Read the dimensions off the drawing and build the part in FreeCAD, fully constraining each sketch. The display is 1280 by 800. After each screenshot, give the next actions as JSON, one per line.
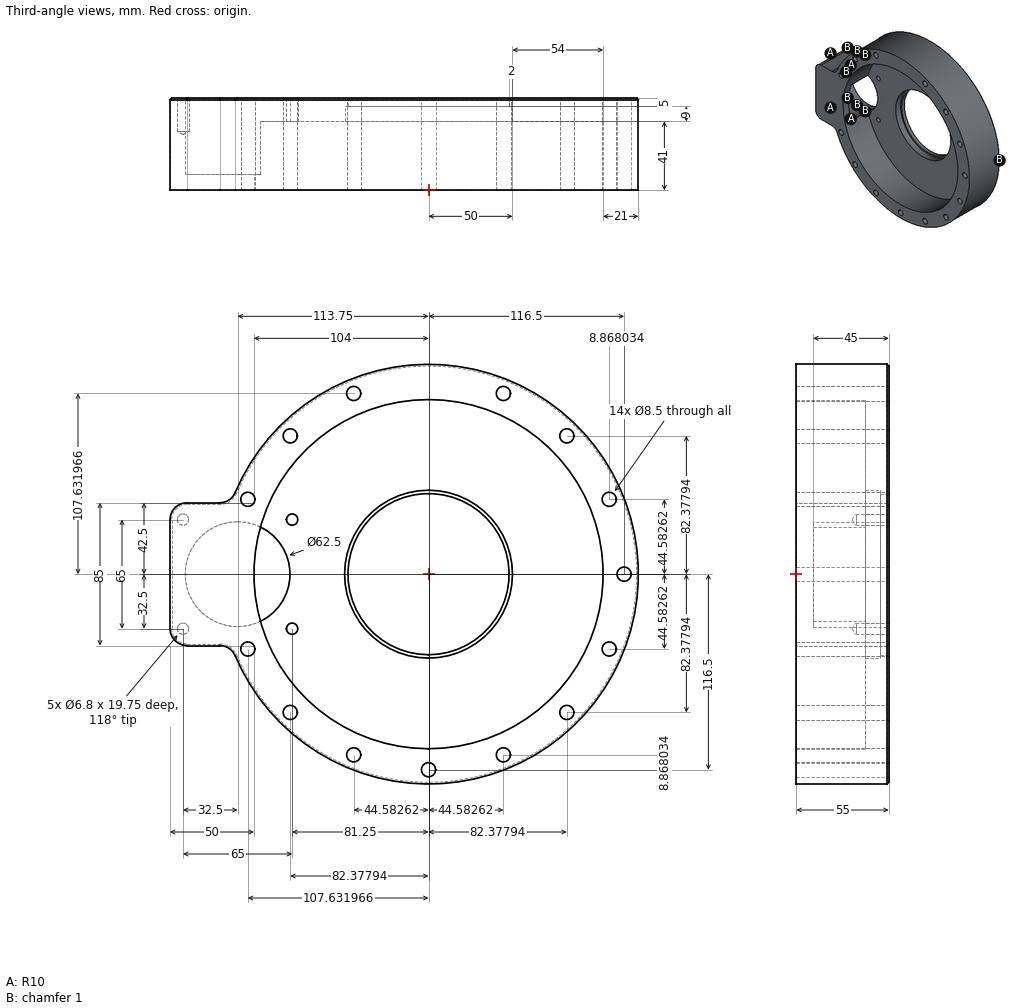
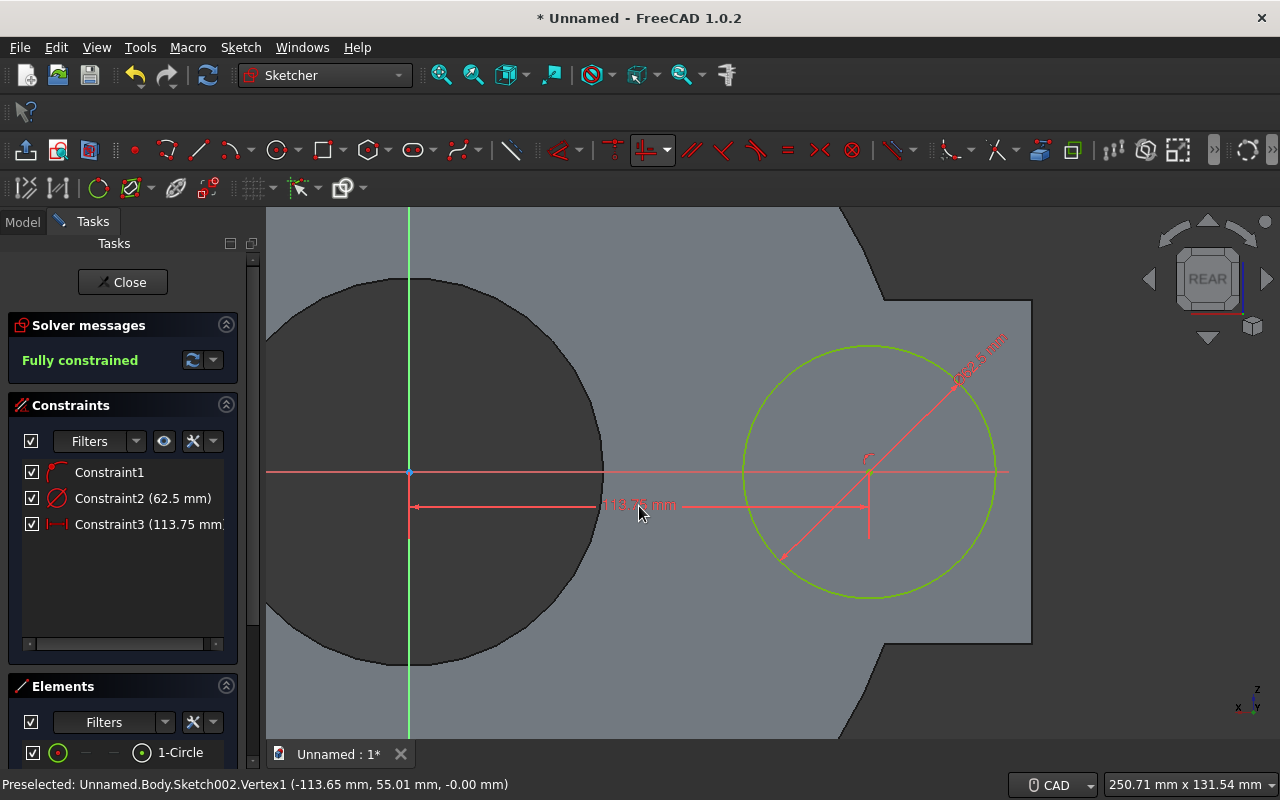
{"action": "left_click", "coordinate": [123, 282]}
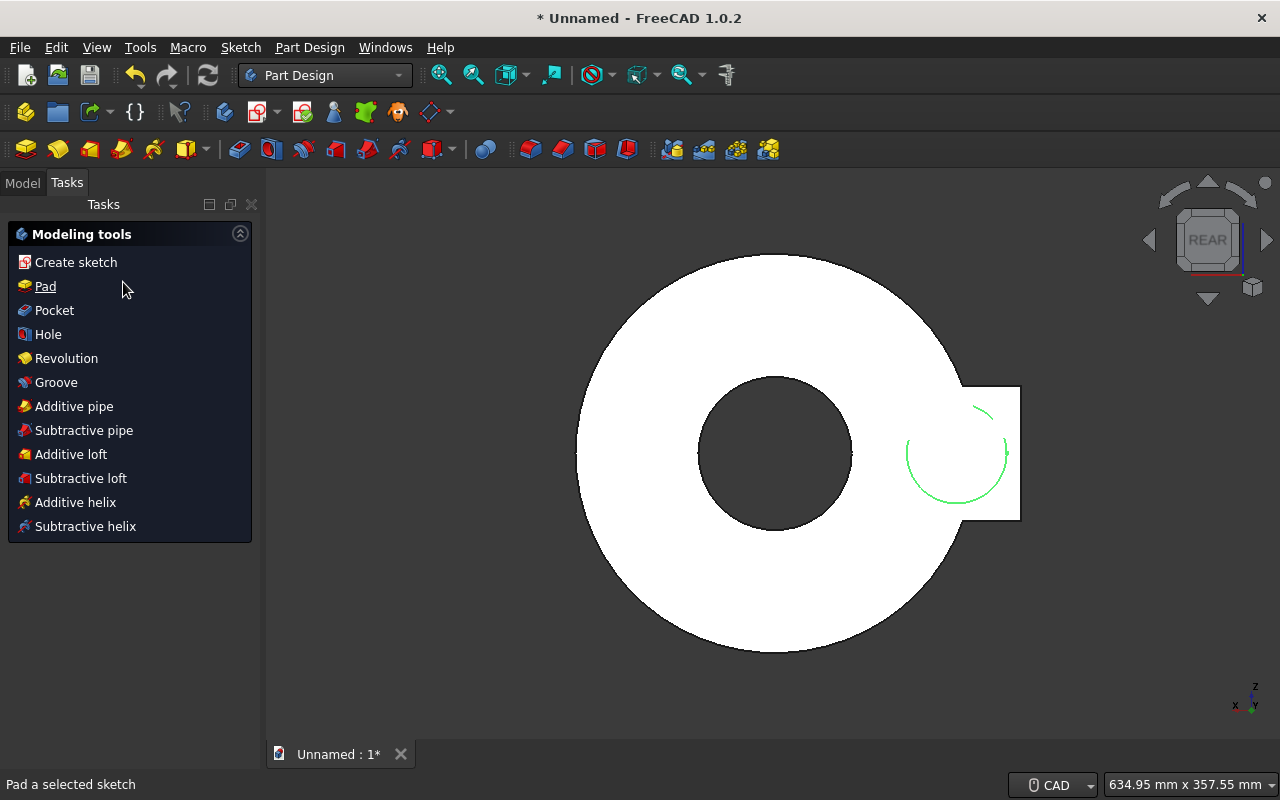
{"action": "left_click", "coordinate": [240, 150]}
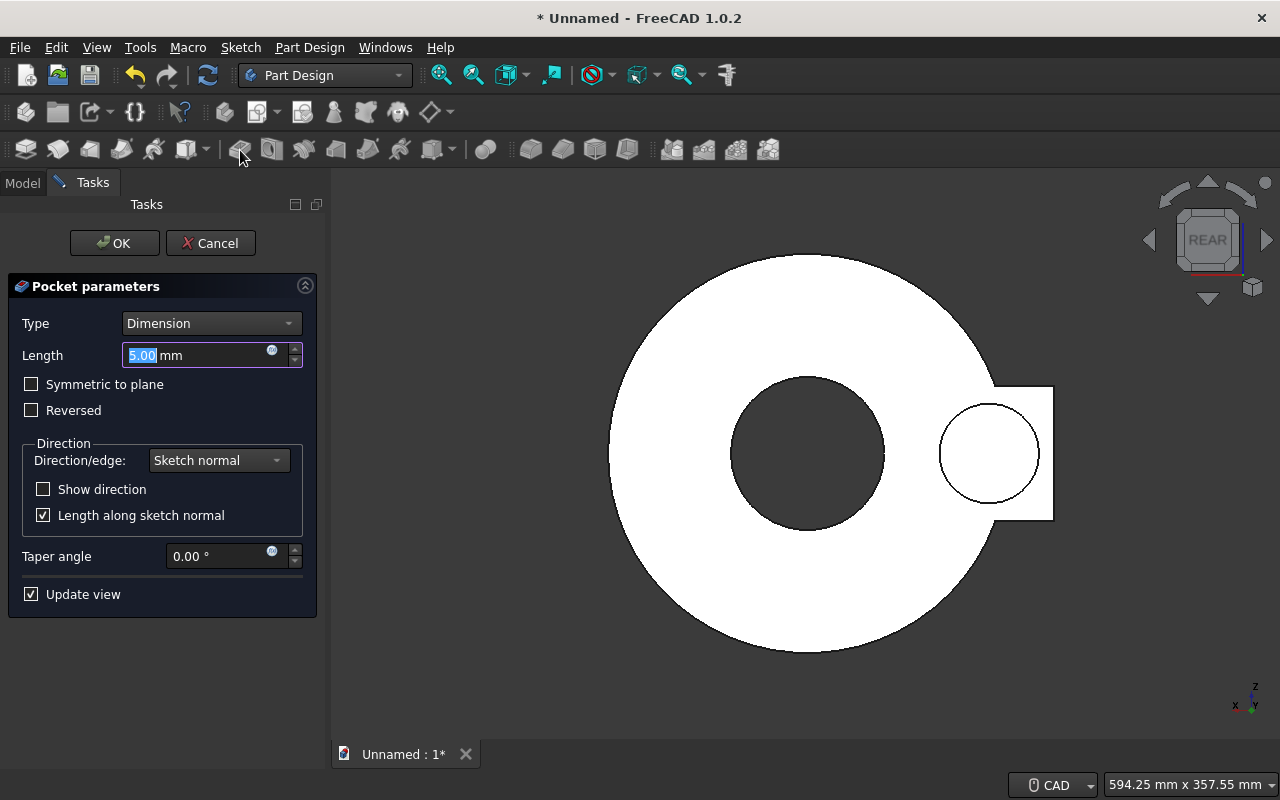
{"action": "type", "text": "45"}
{"action": "key", "text": "Tab"}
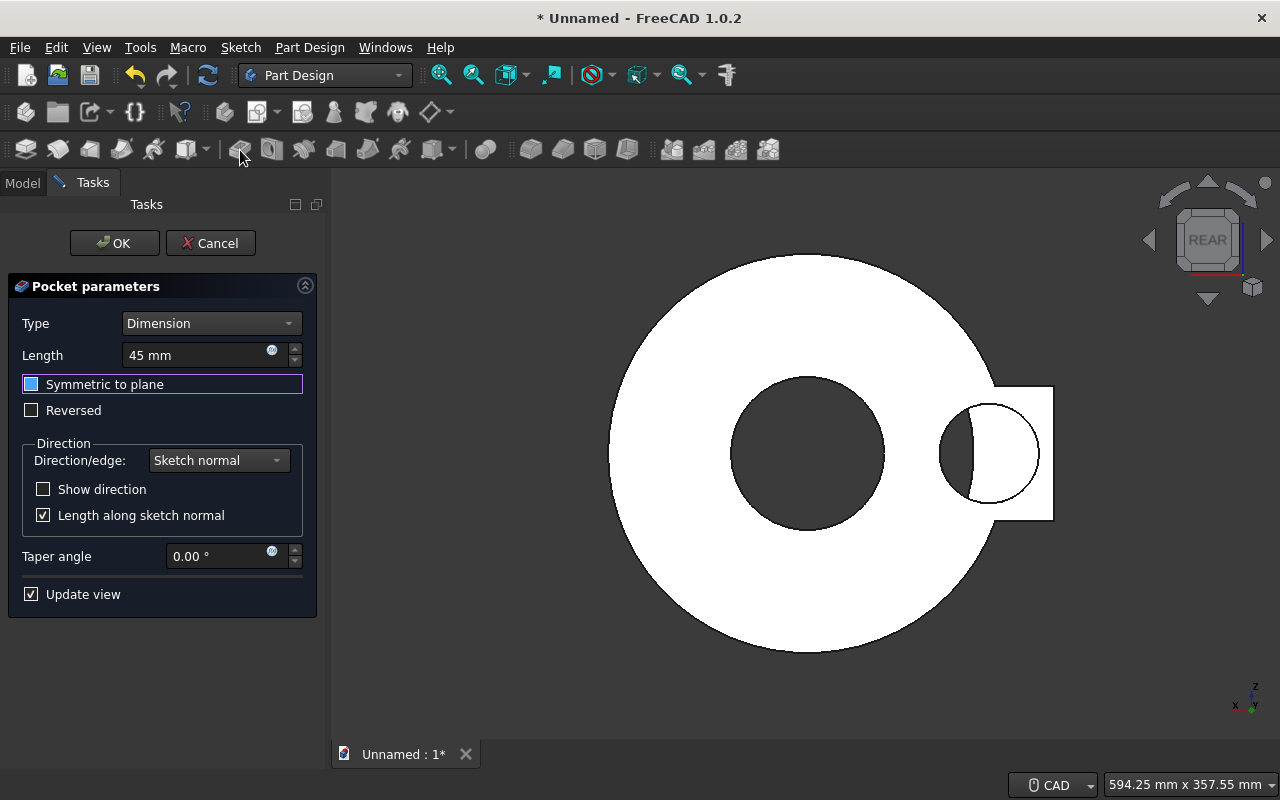
{"action": "left_click", "coordinate": [115, 243]}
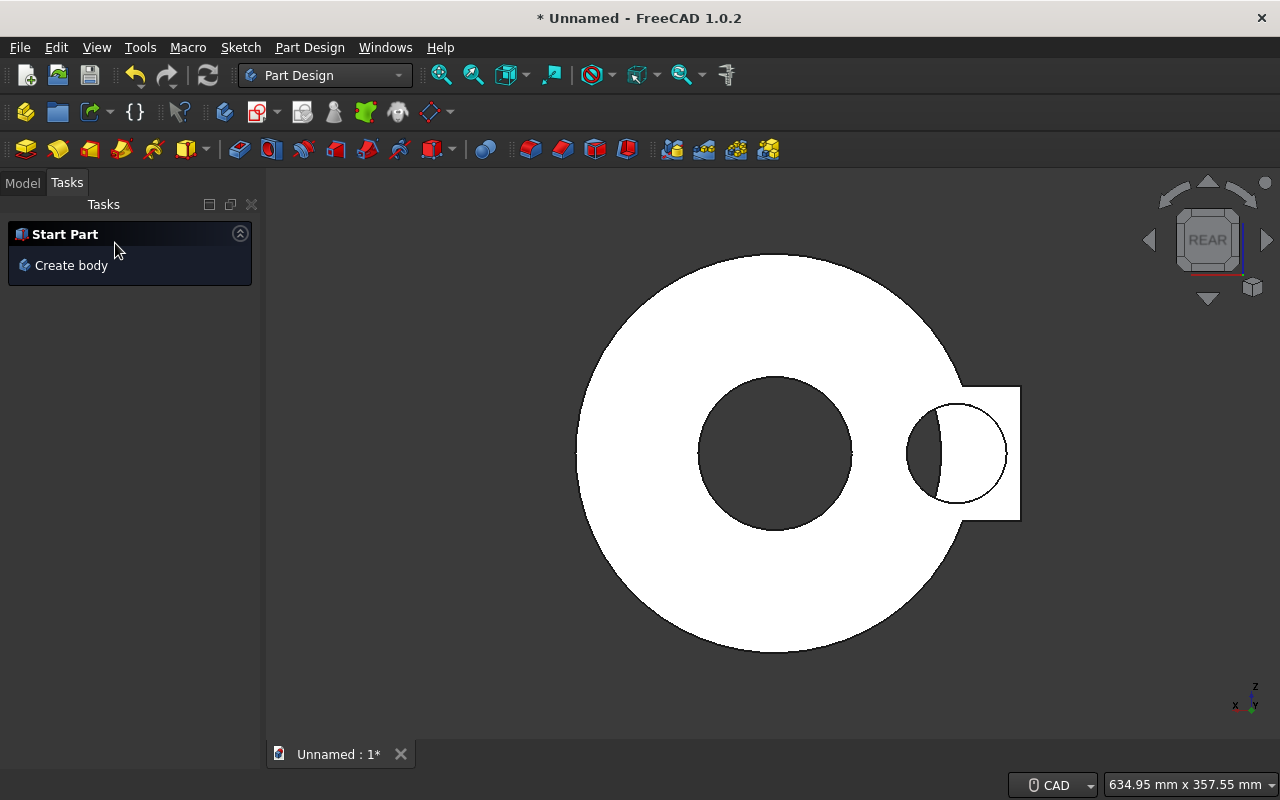
{"action": "left_click", "coordinate": [862, 338]}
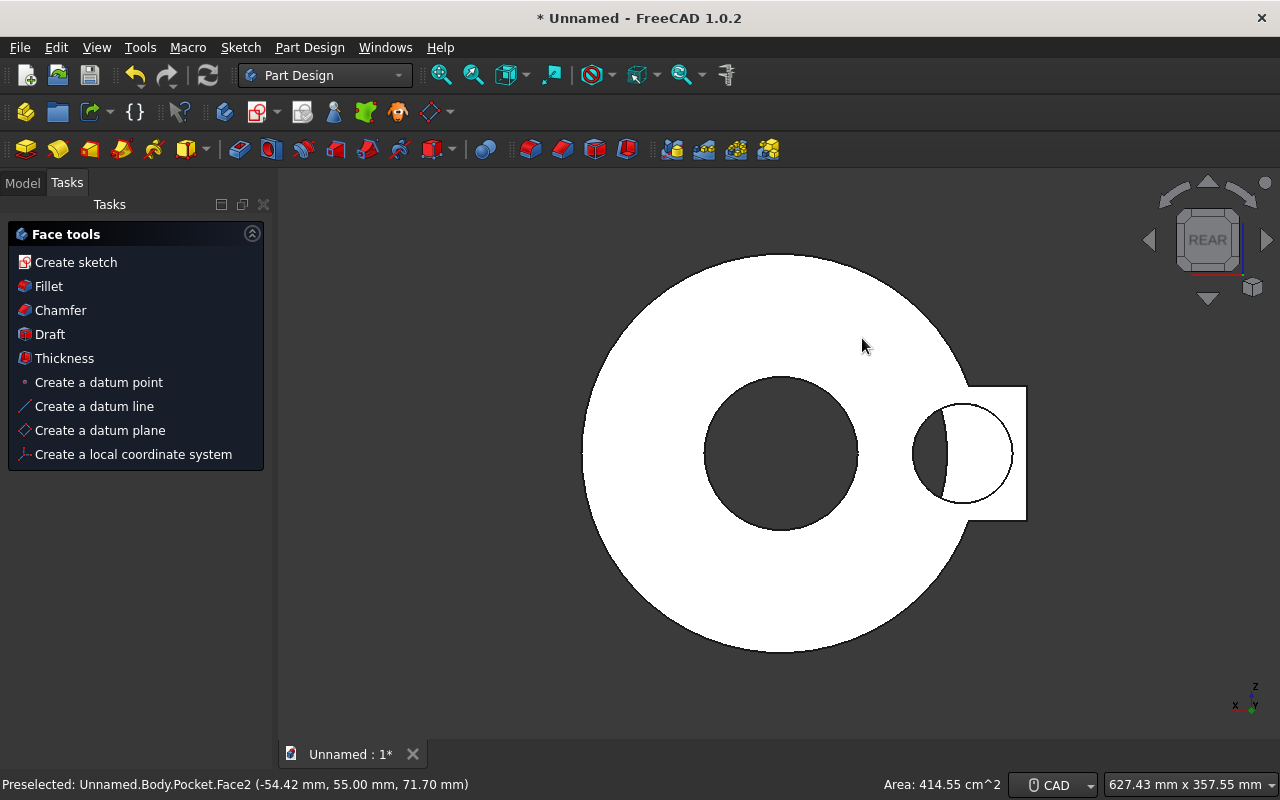
{"action": "left_click", "coordinate": [258, 112]}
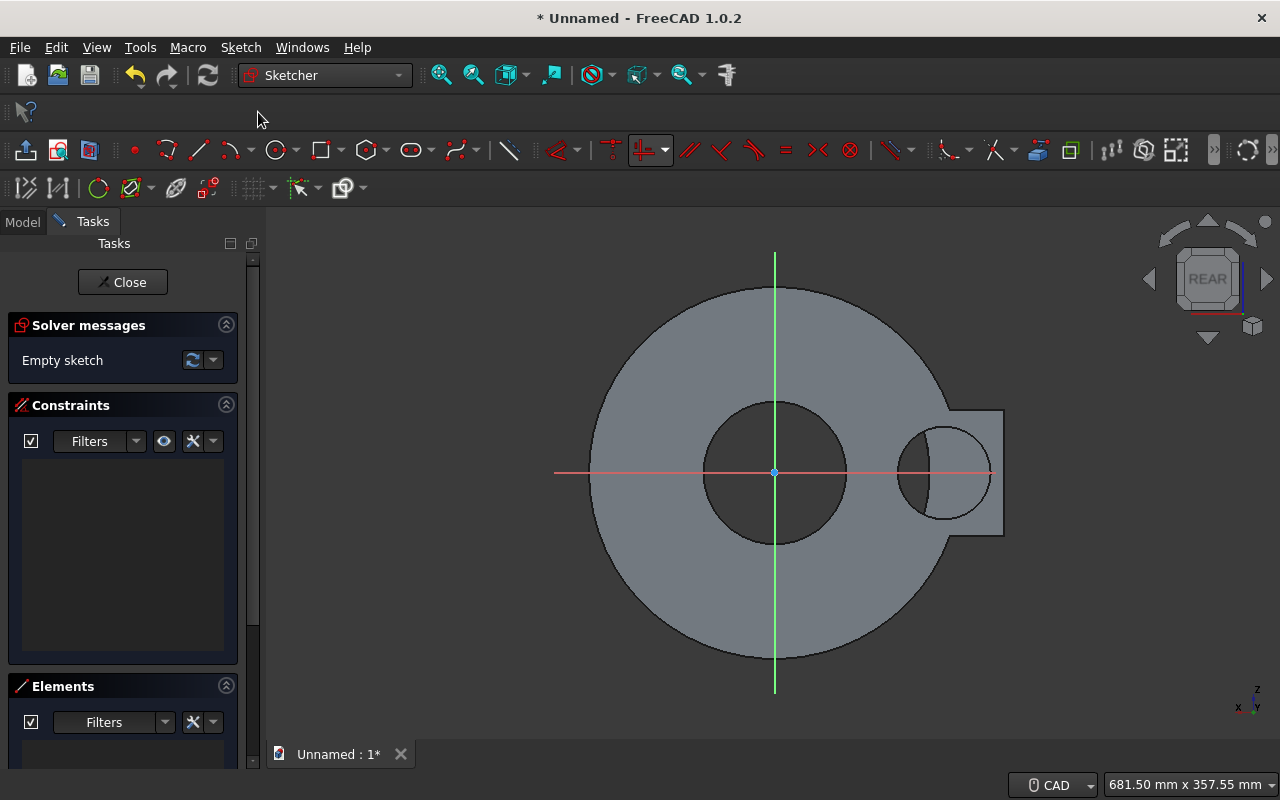
{"action": "scroll", "coordinate": [992, 473], "scroll_direction": "up", "scroll_amount": 5}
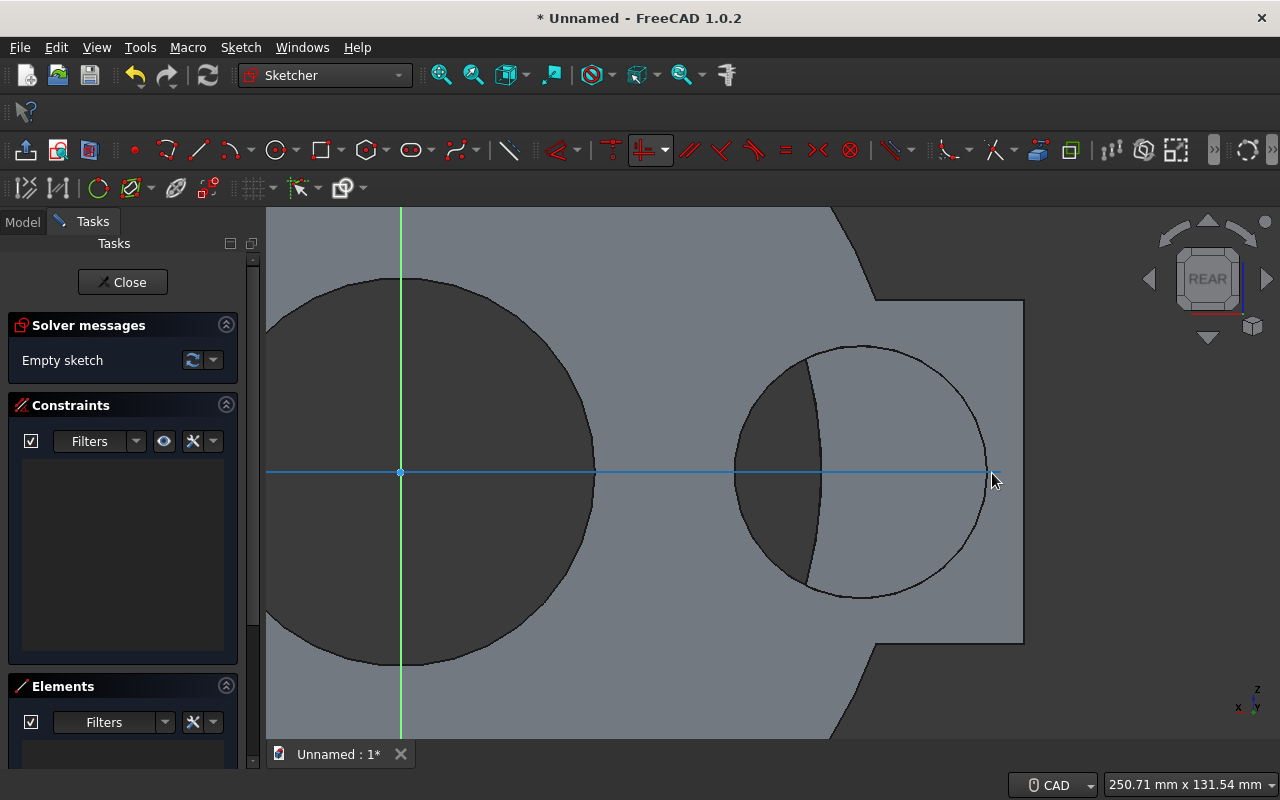
{"action": "left_click", "coordinate": [276, 150]}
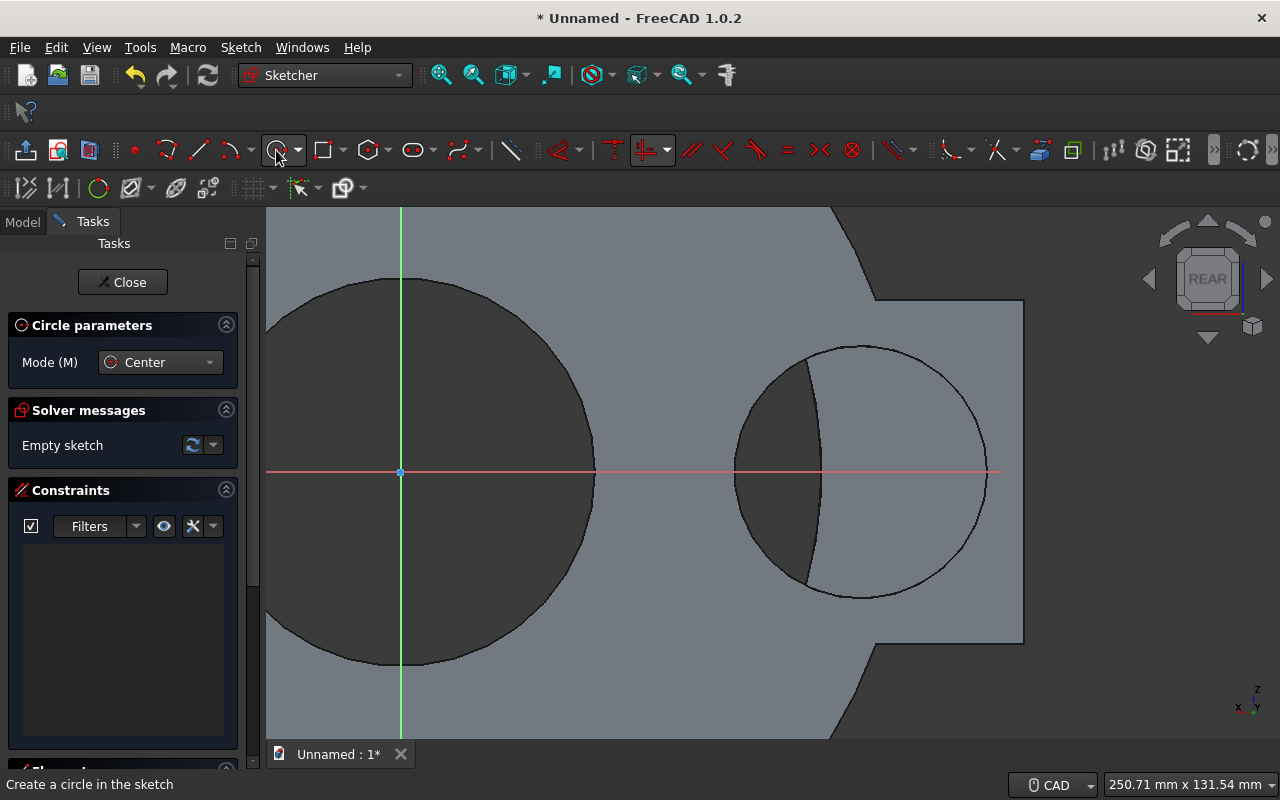
{"action": "scroll", "coordinate": [992, 604], "scroll_direction": "up", "scroll_amount": 3}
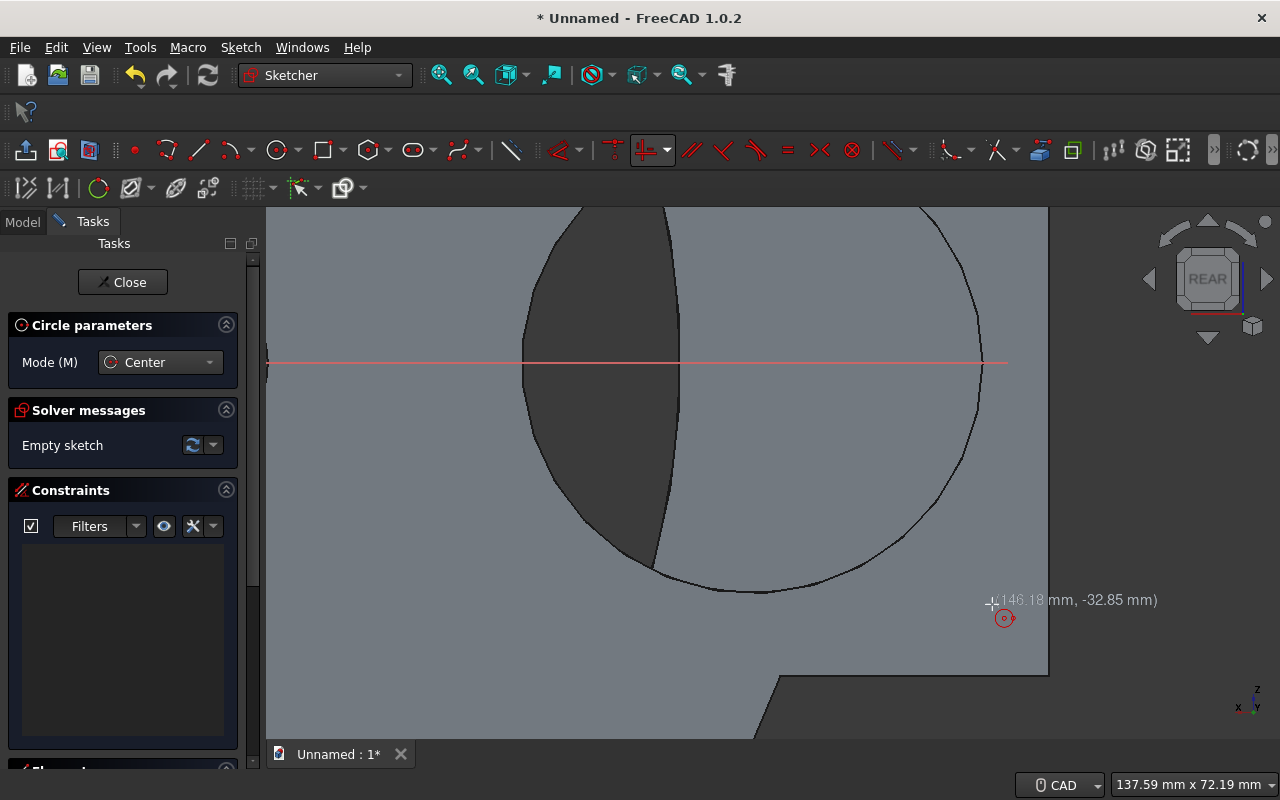
{"action": "left_click", "coordinate": [992, 603]}
{"action": "left_click", "coordinate": [1010, 585]}